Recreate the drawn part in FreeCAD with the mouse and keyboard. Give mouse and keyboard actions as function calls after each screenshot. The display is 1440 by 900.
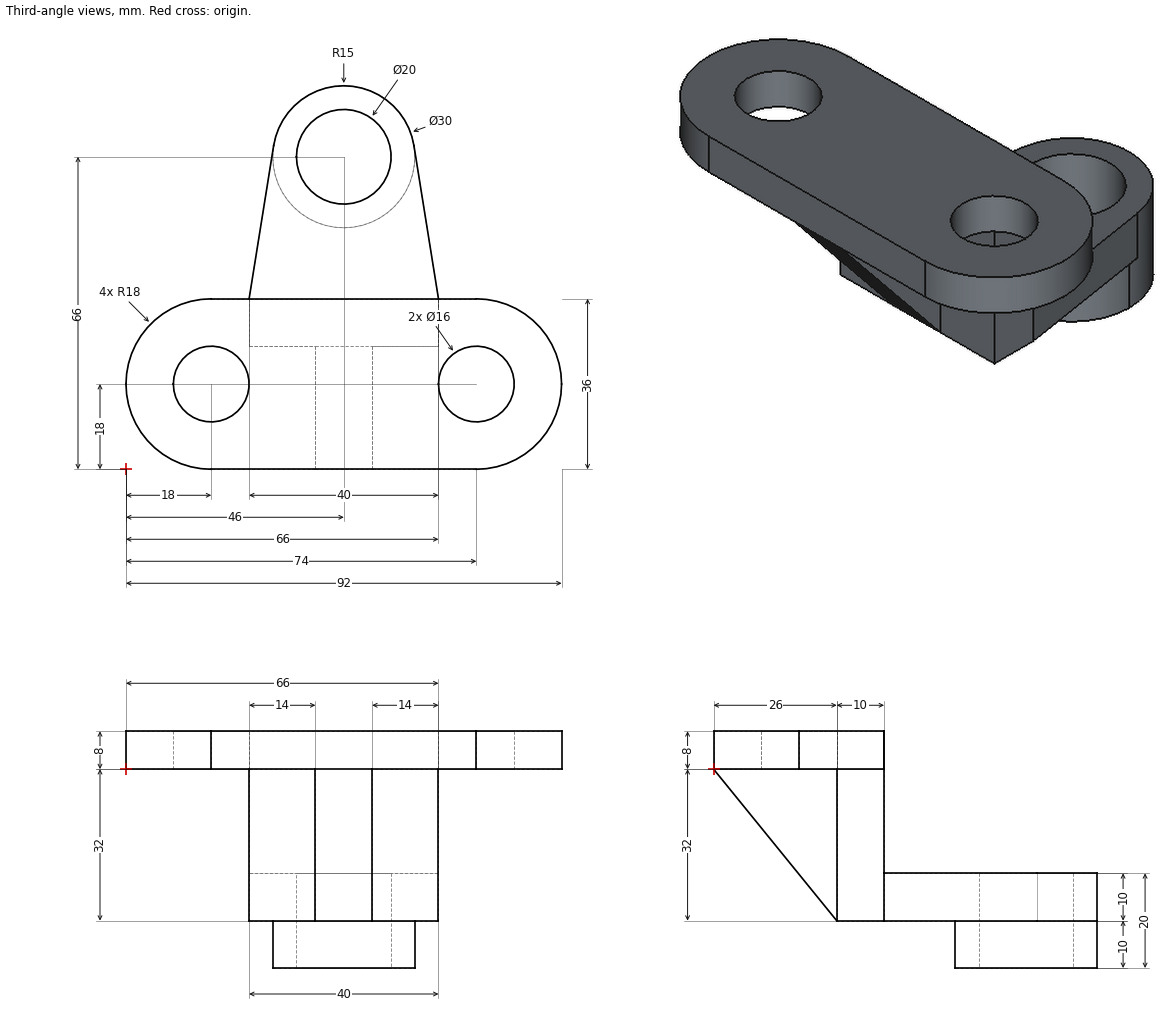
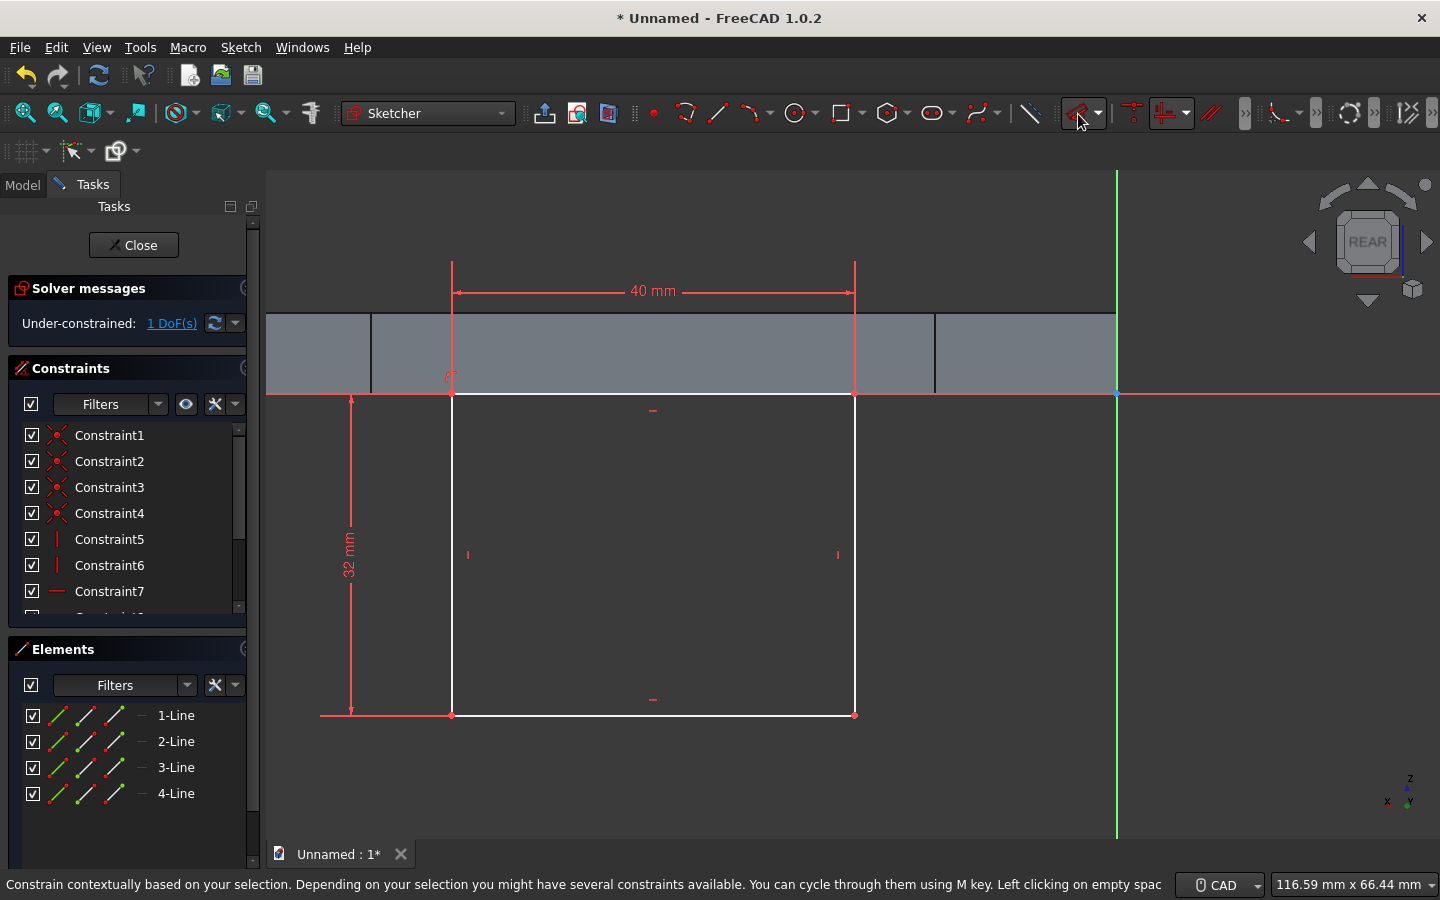
click(452, 394)
click(784, 360)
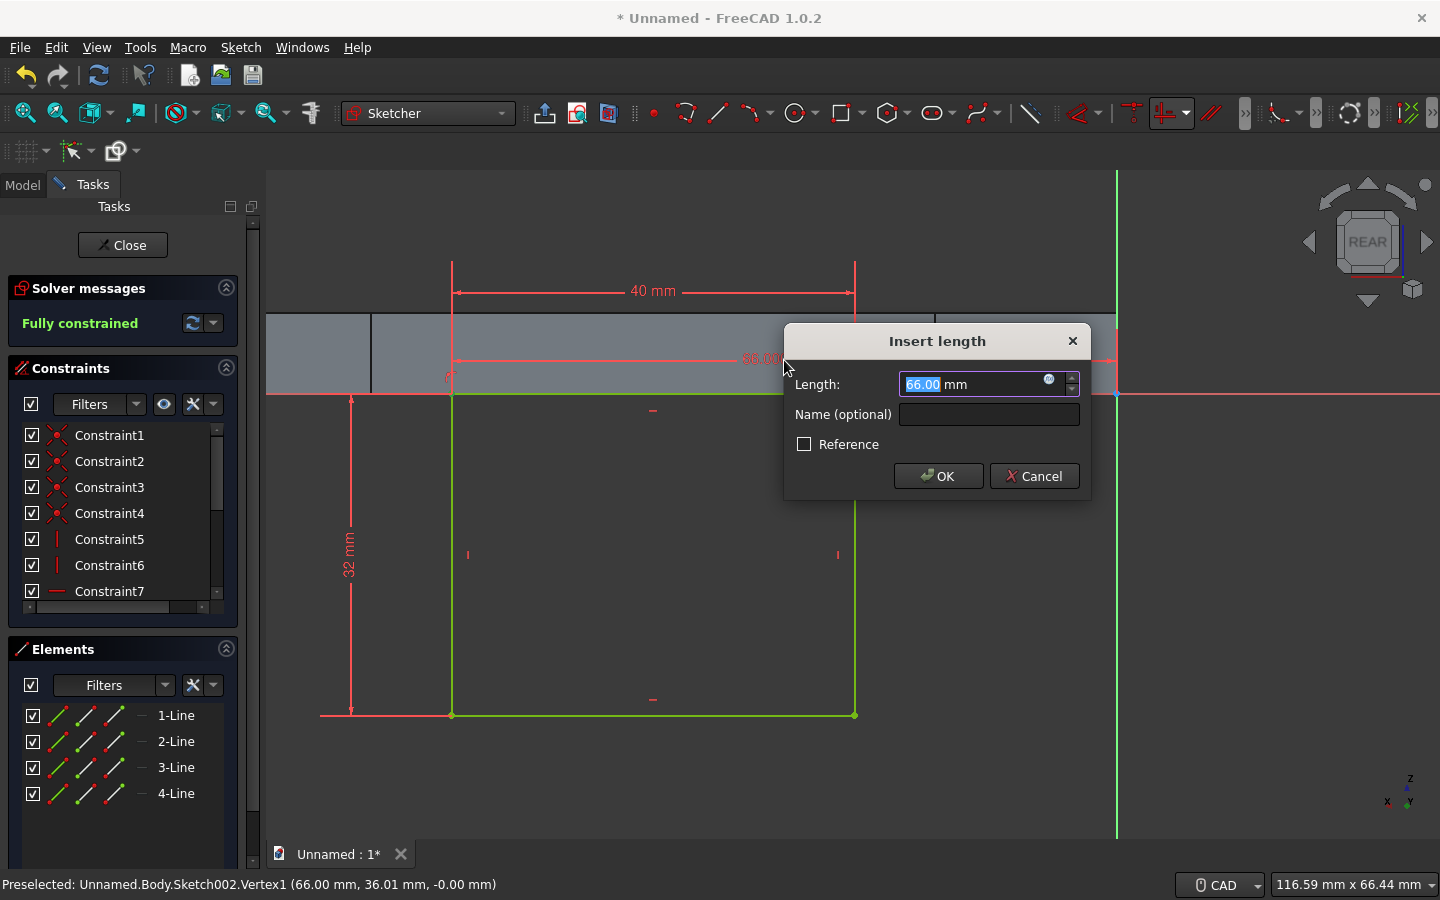
text(66)
key(Return)
key(Escape)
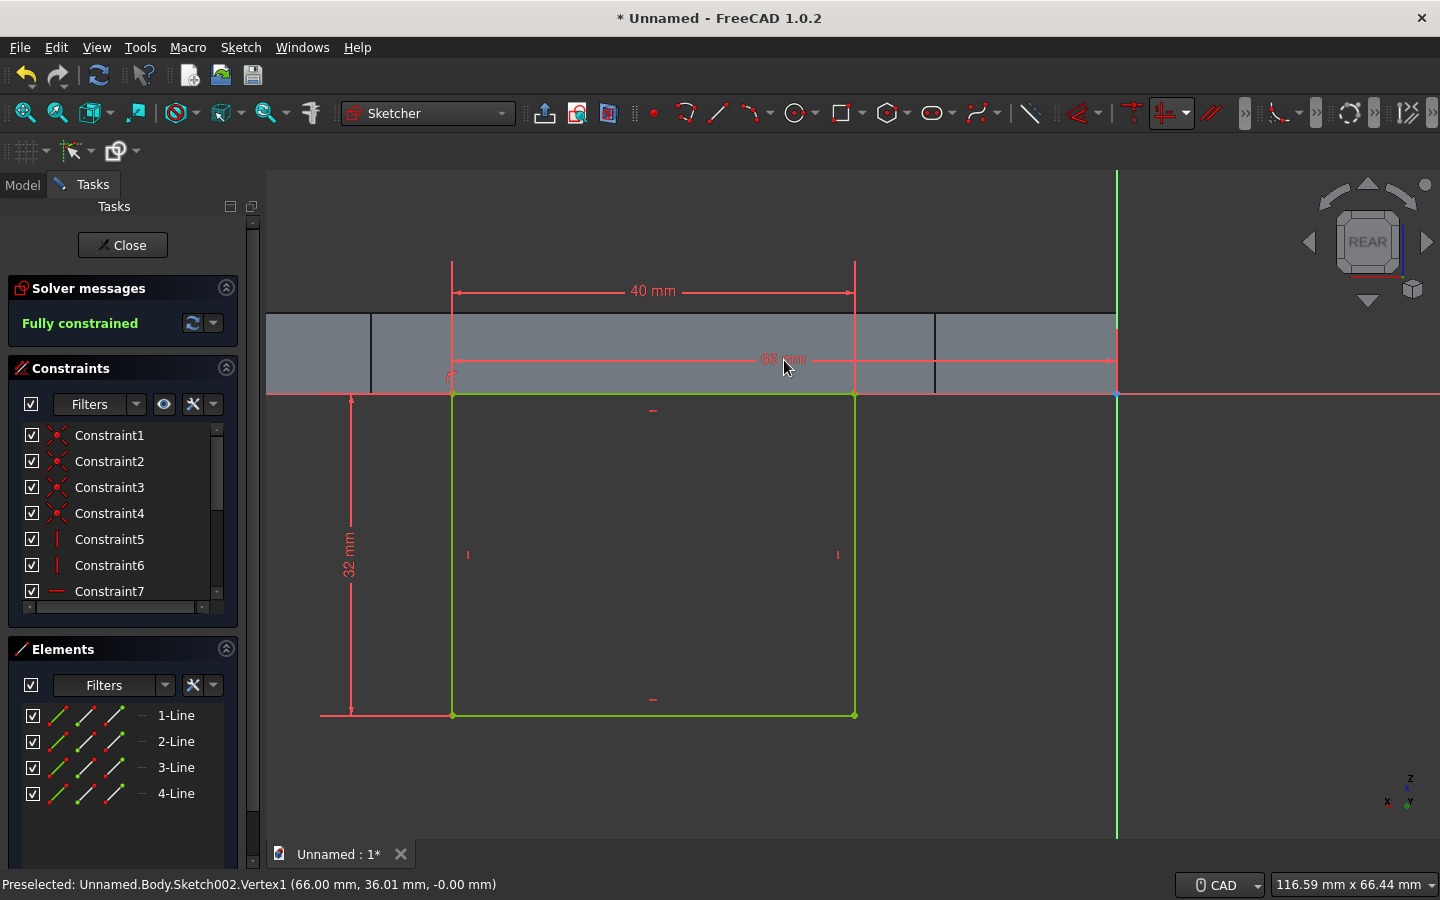
click(123, 245)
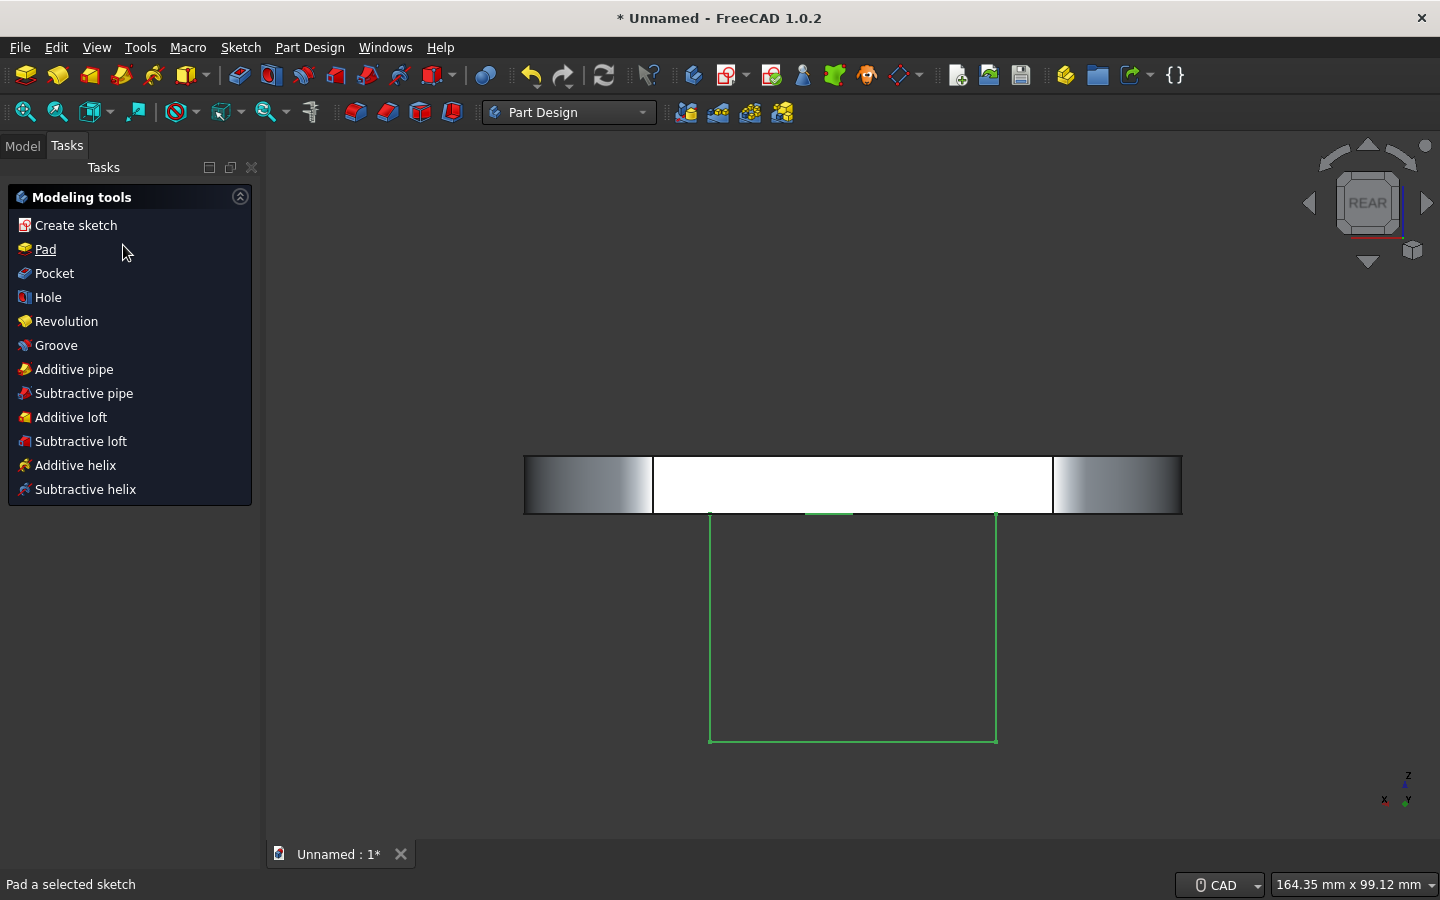
click(26, 76)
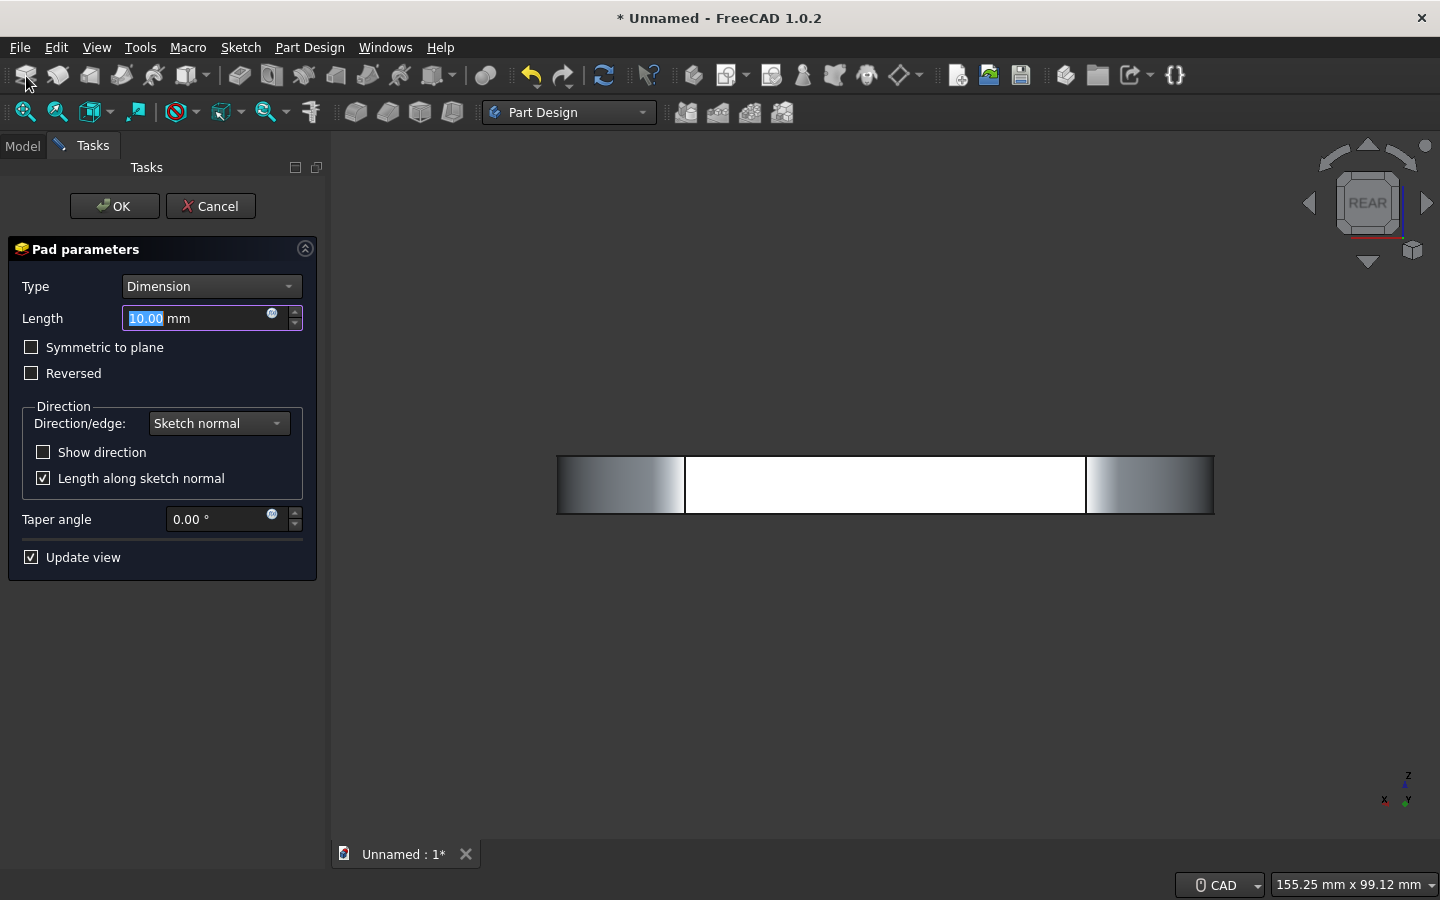
text(10)
key(Tab)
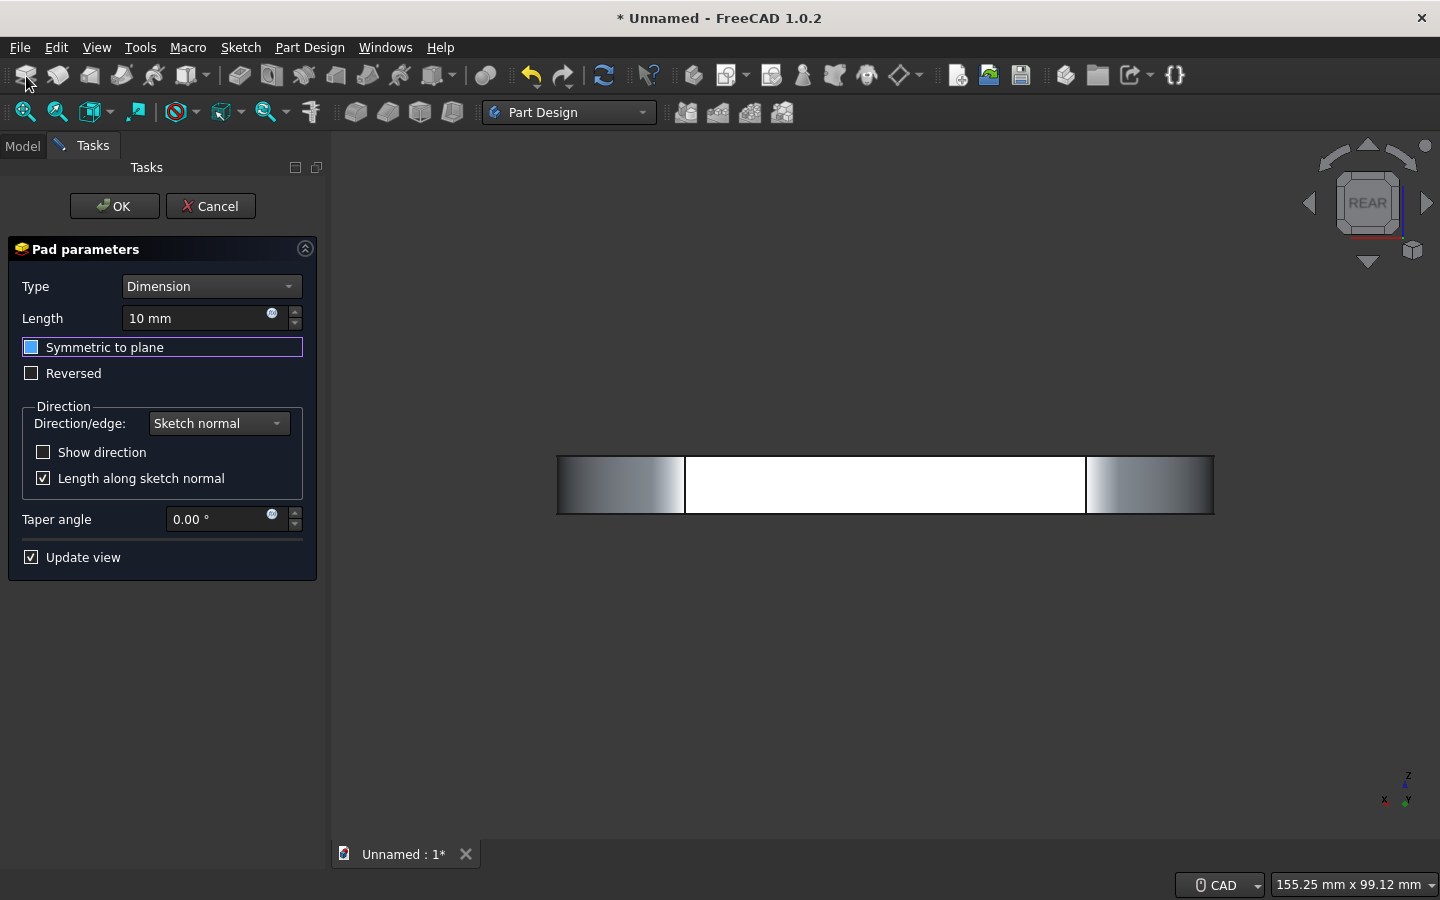
click(30, 373)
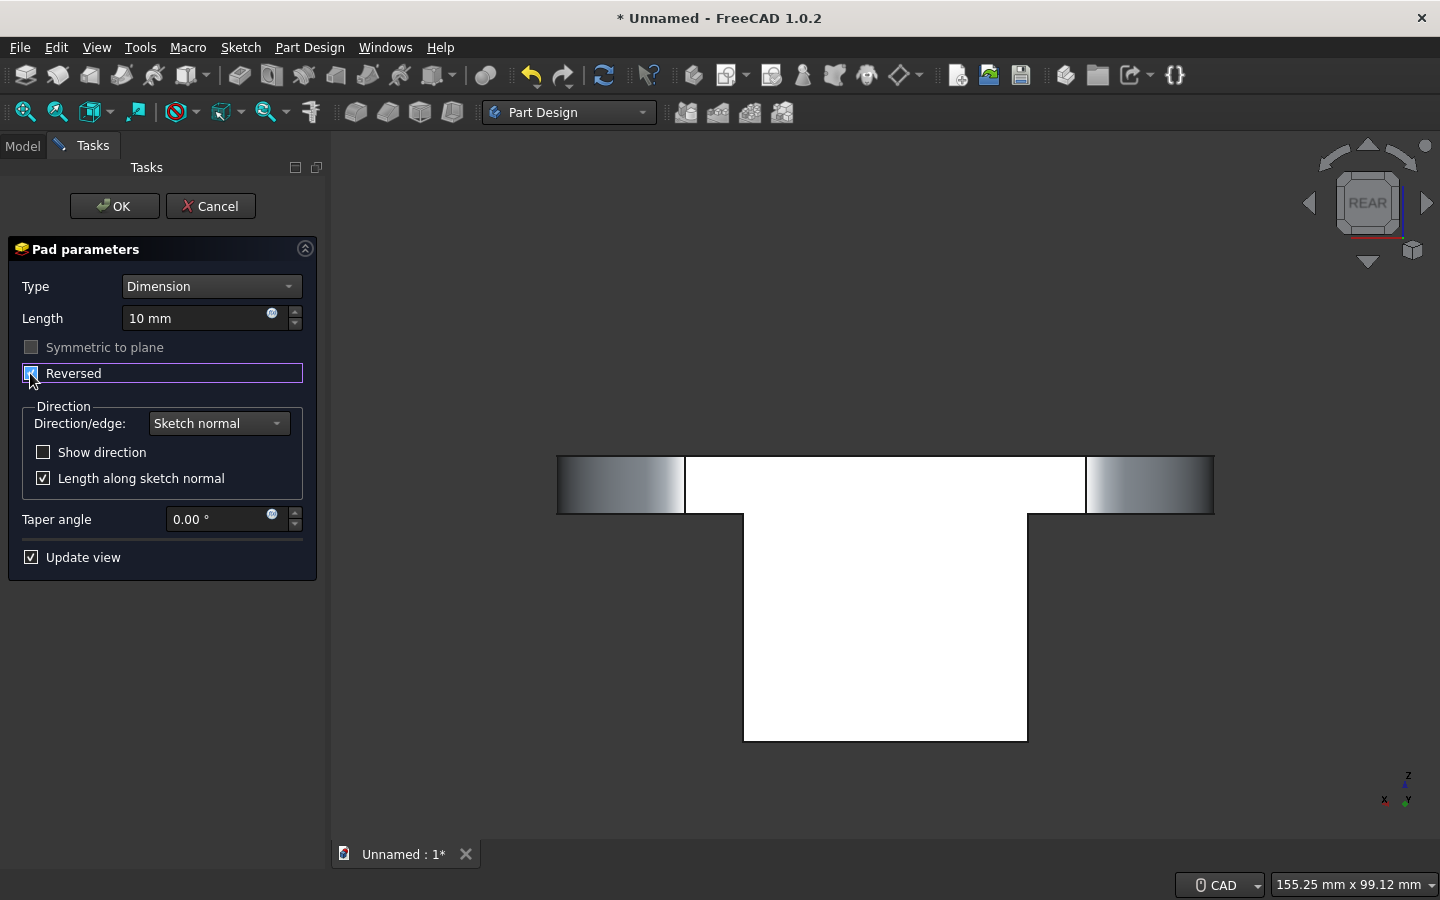
click(115, 206)